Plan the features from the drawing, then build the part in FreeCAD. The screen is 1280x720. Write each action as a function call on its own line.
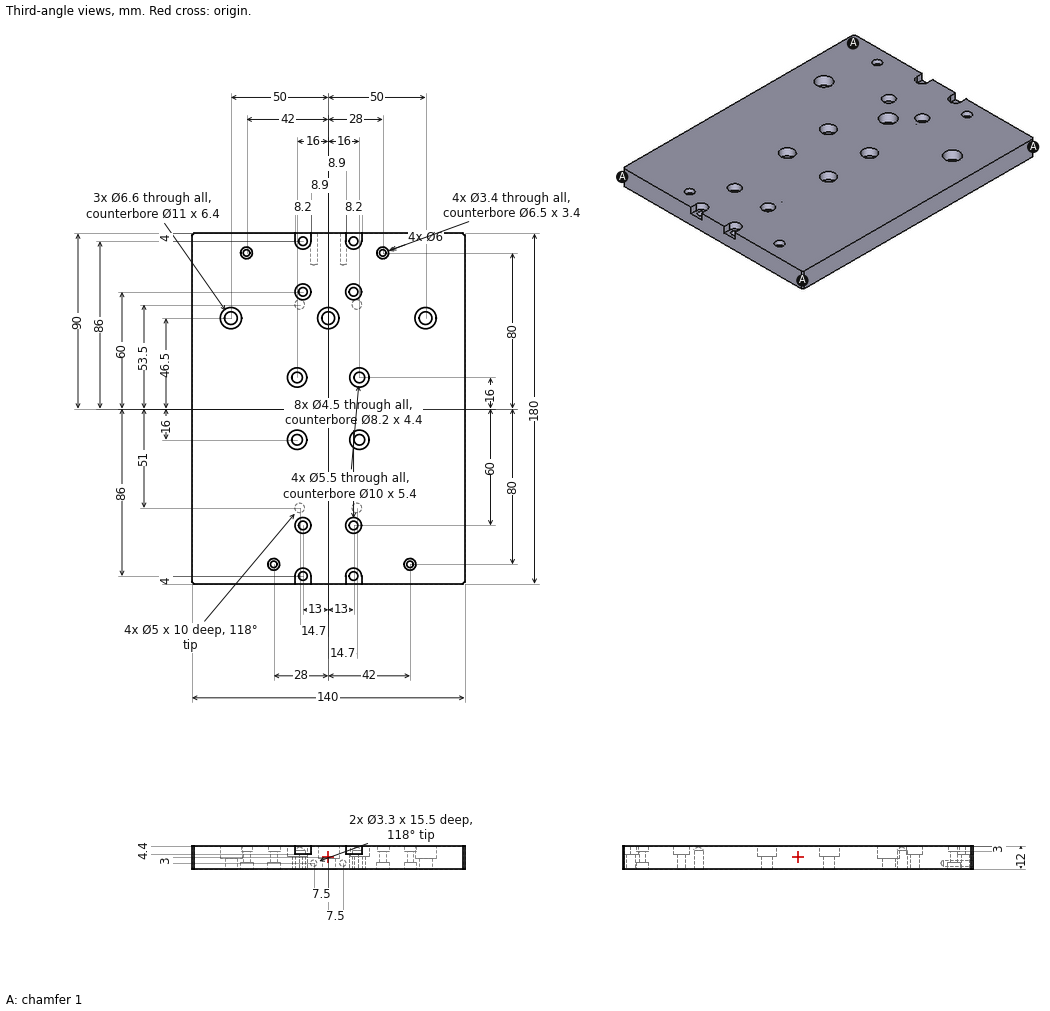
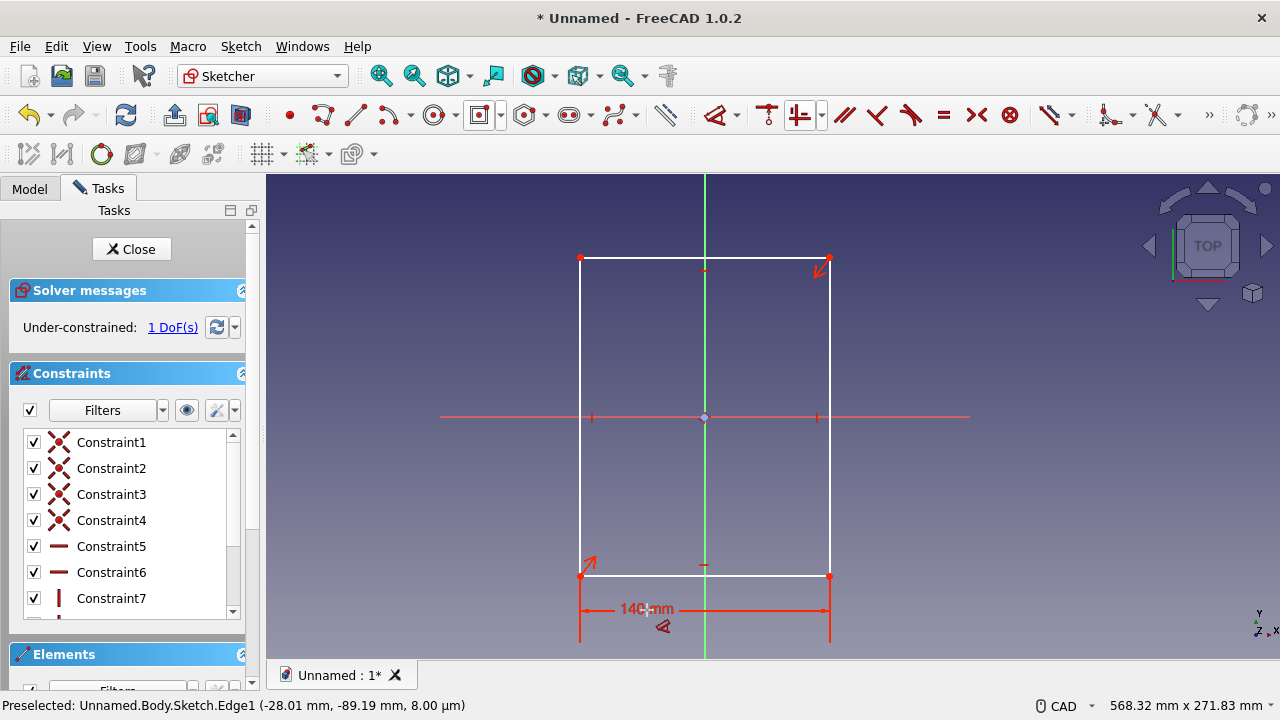
click(830, 481)
click(864, 344)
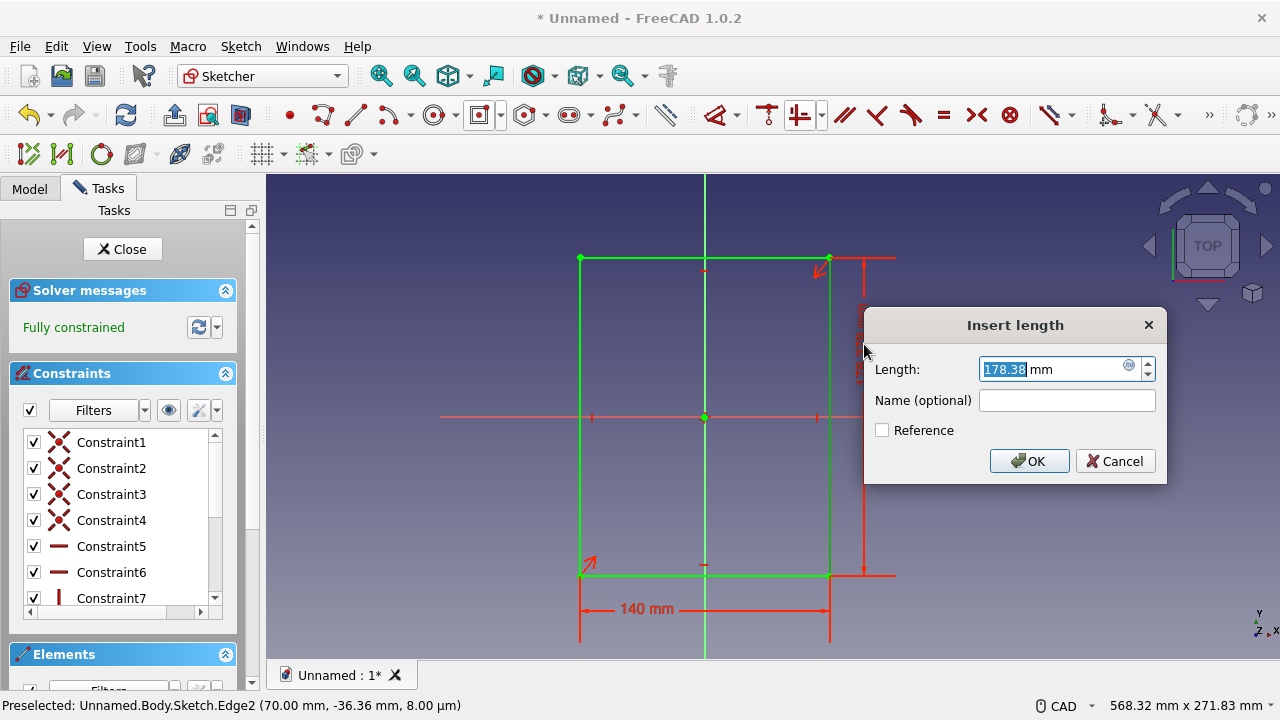
text(180)
key(Return)
key(Escape)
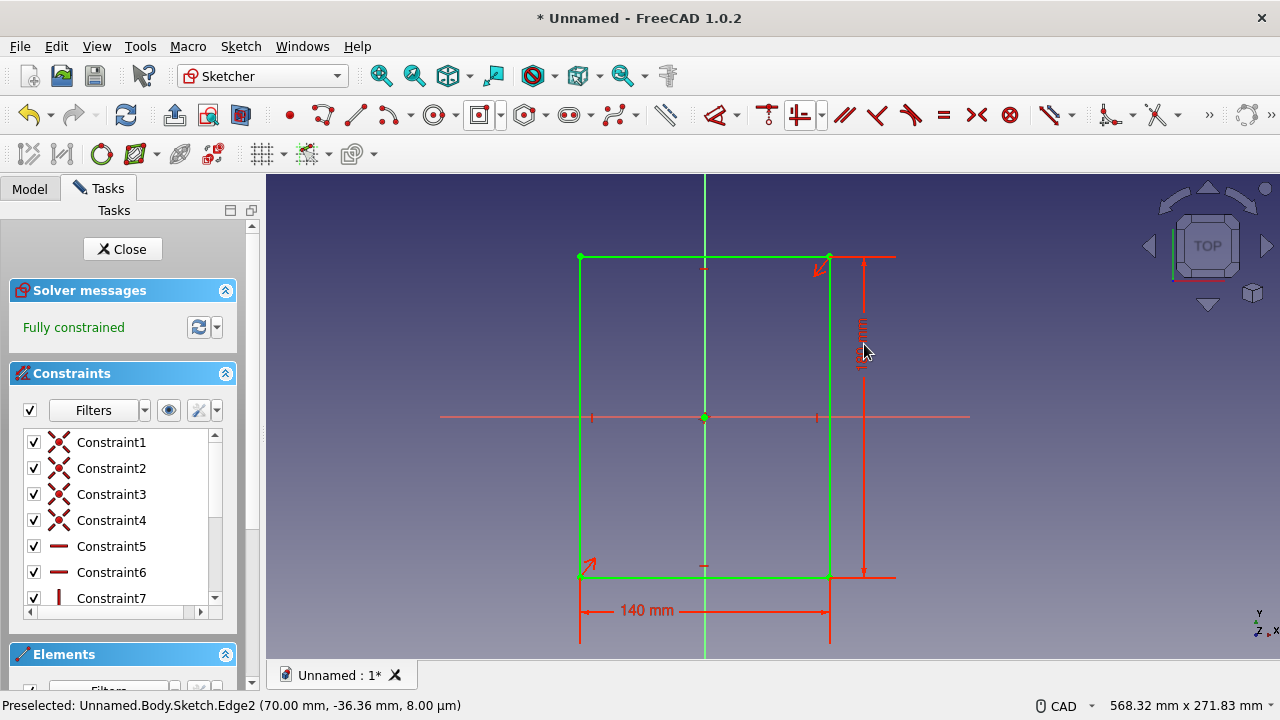
click(123, 249)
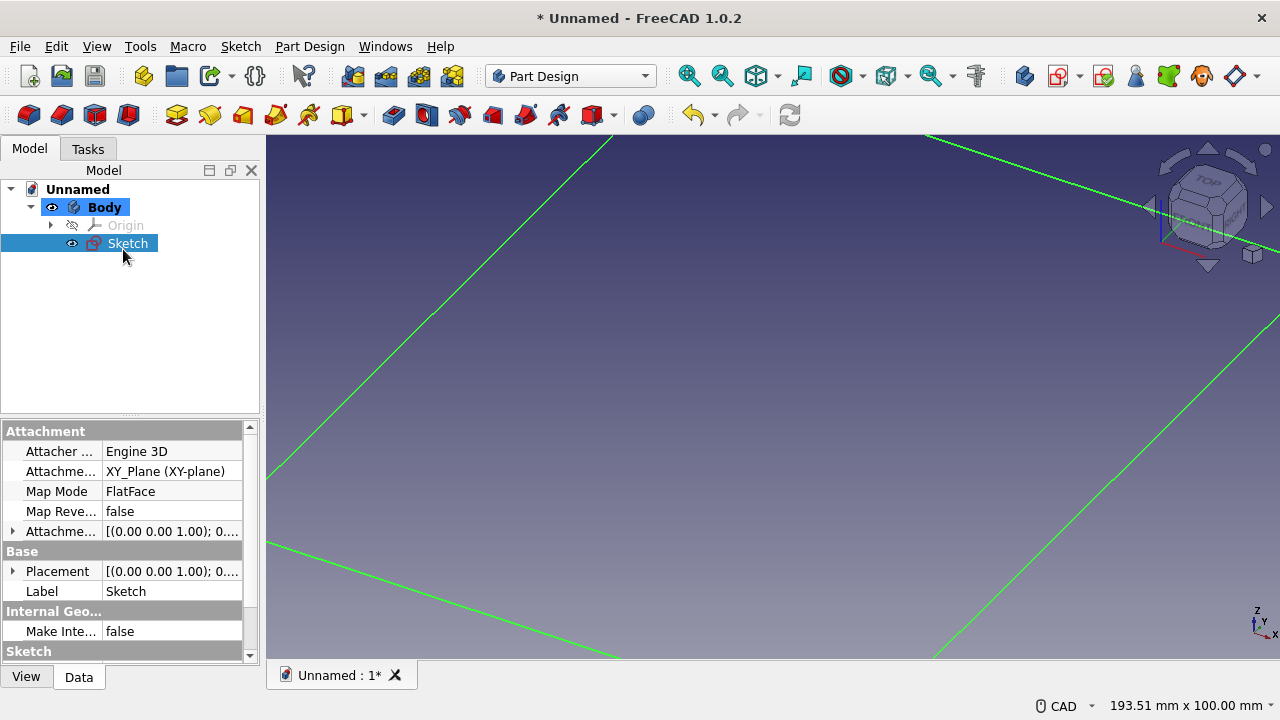
click(177, 116)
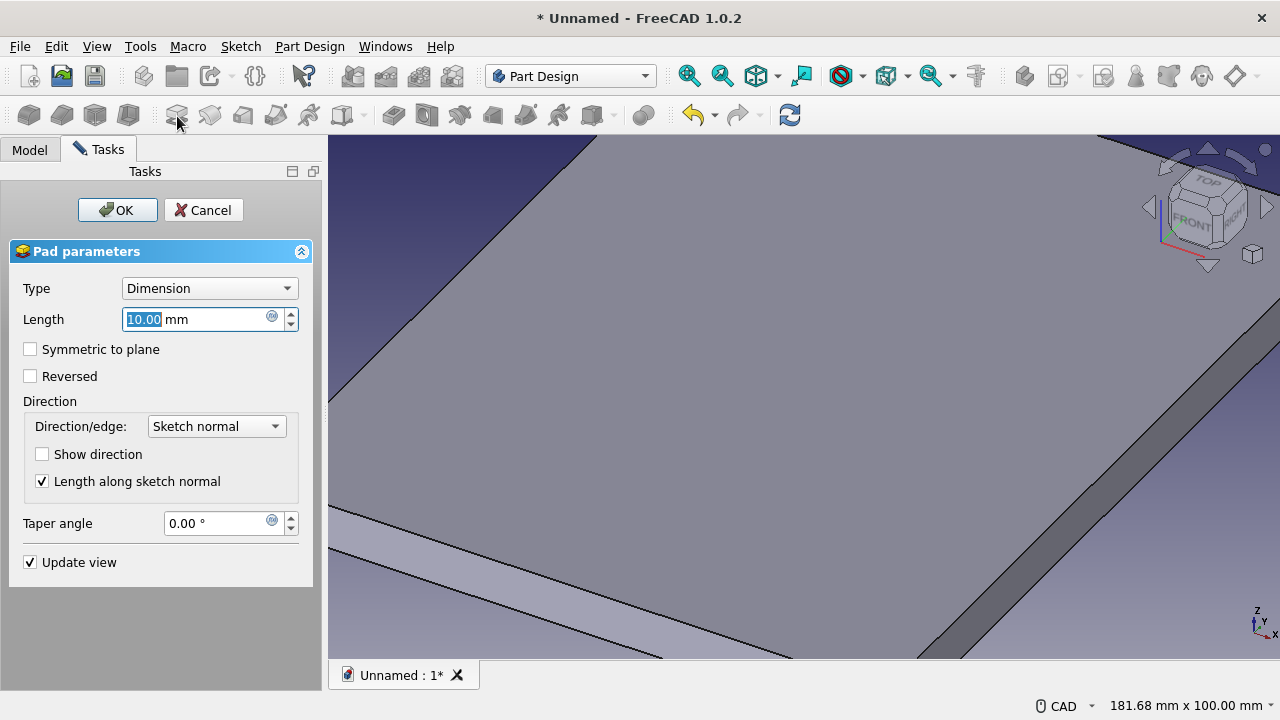
text(12)
key(Tab)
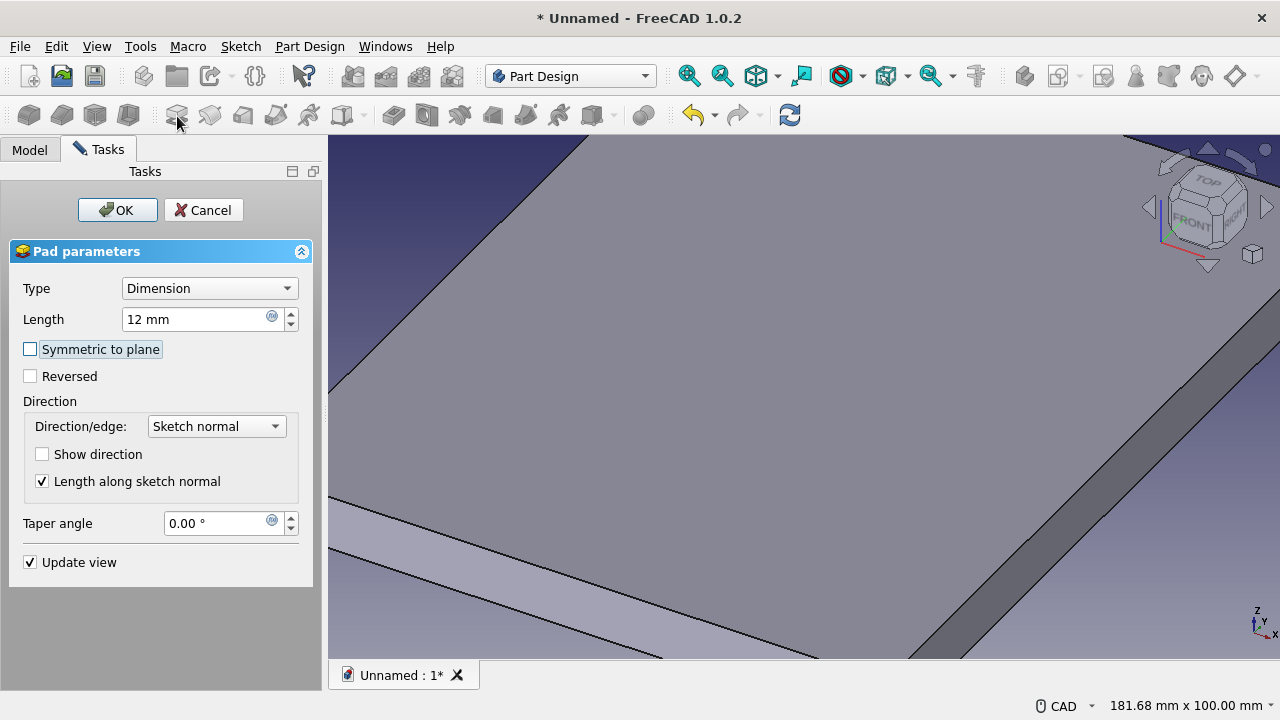
click(31, 349)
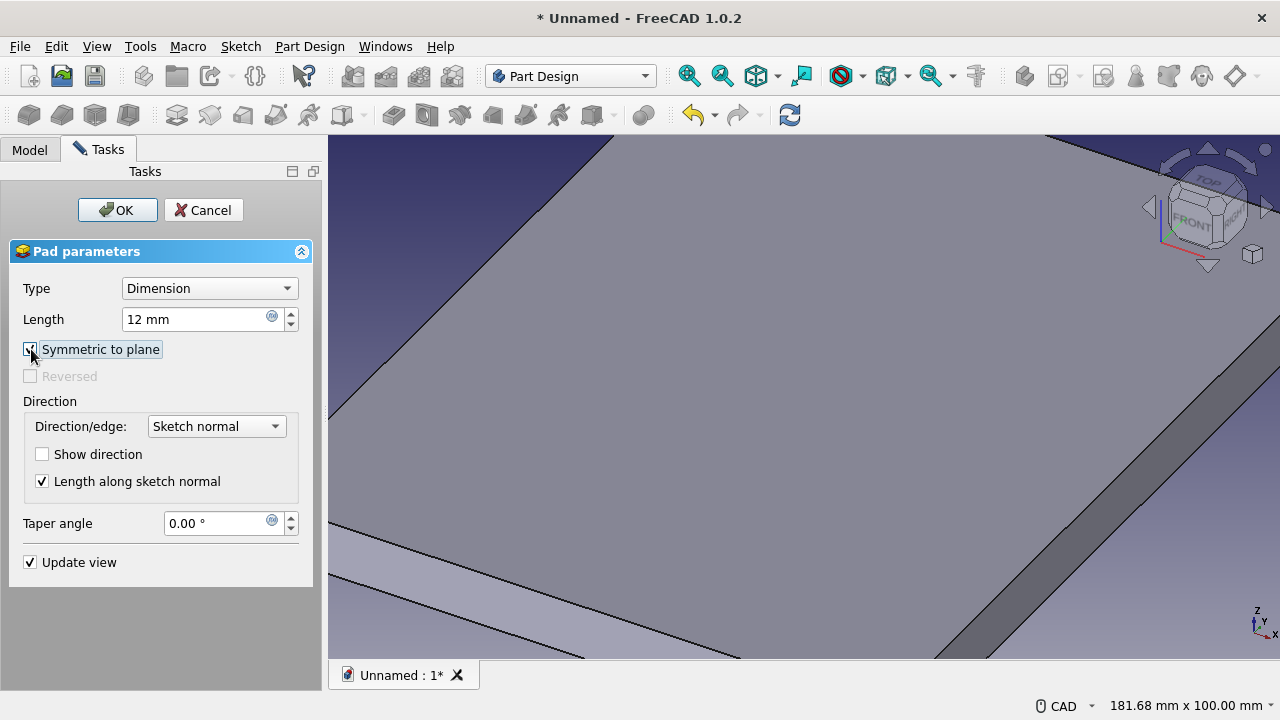
click(118, 210)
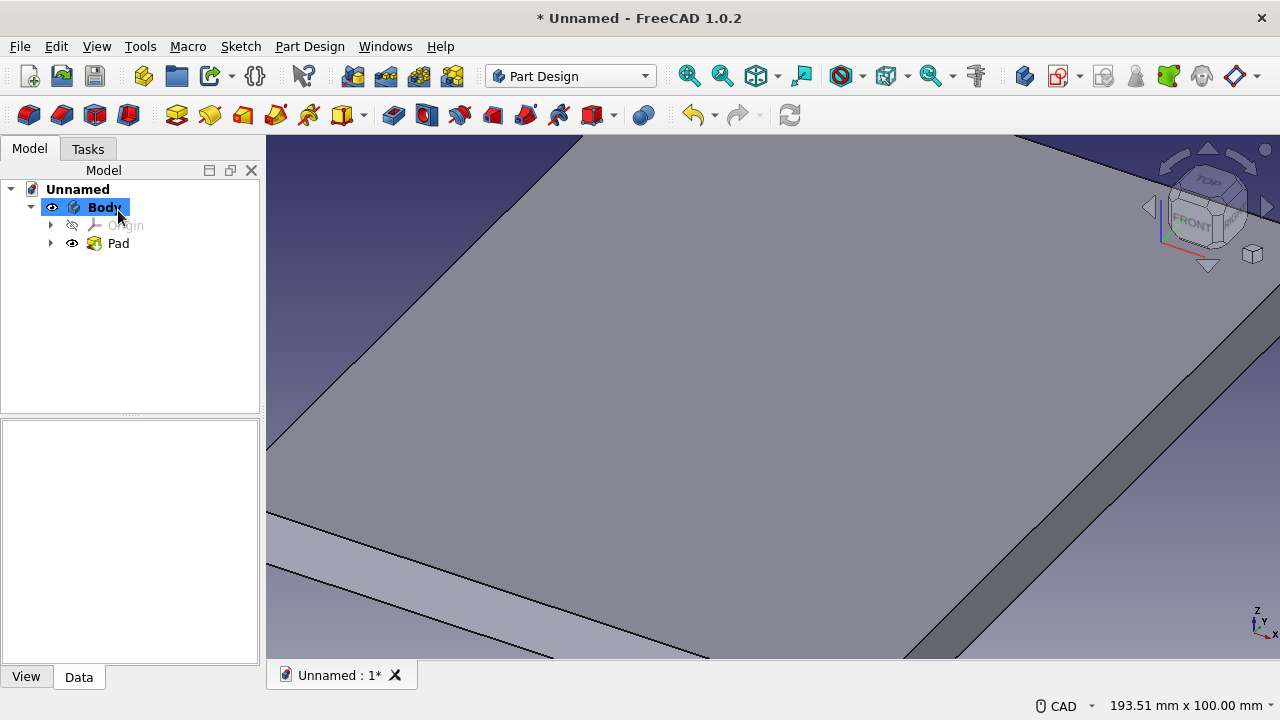
click(690, 76)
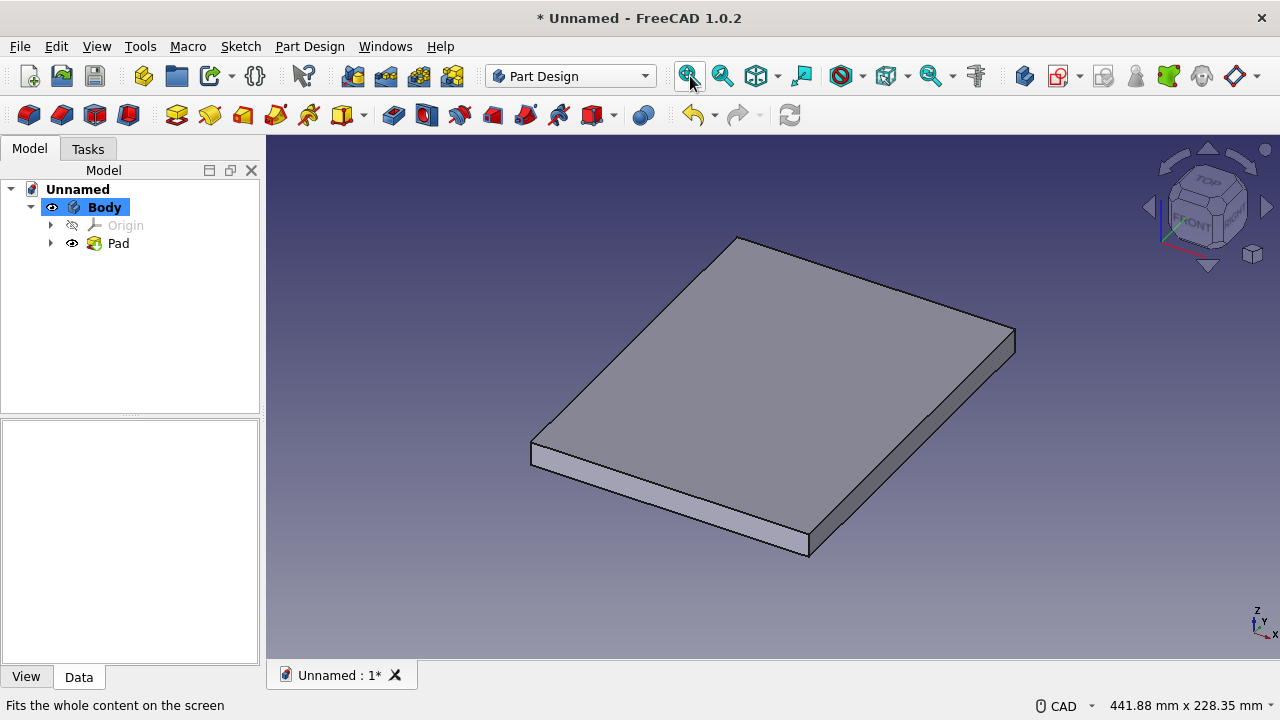
click(773, 385)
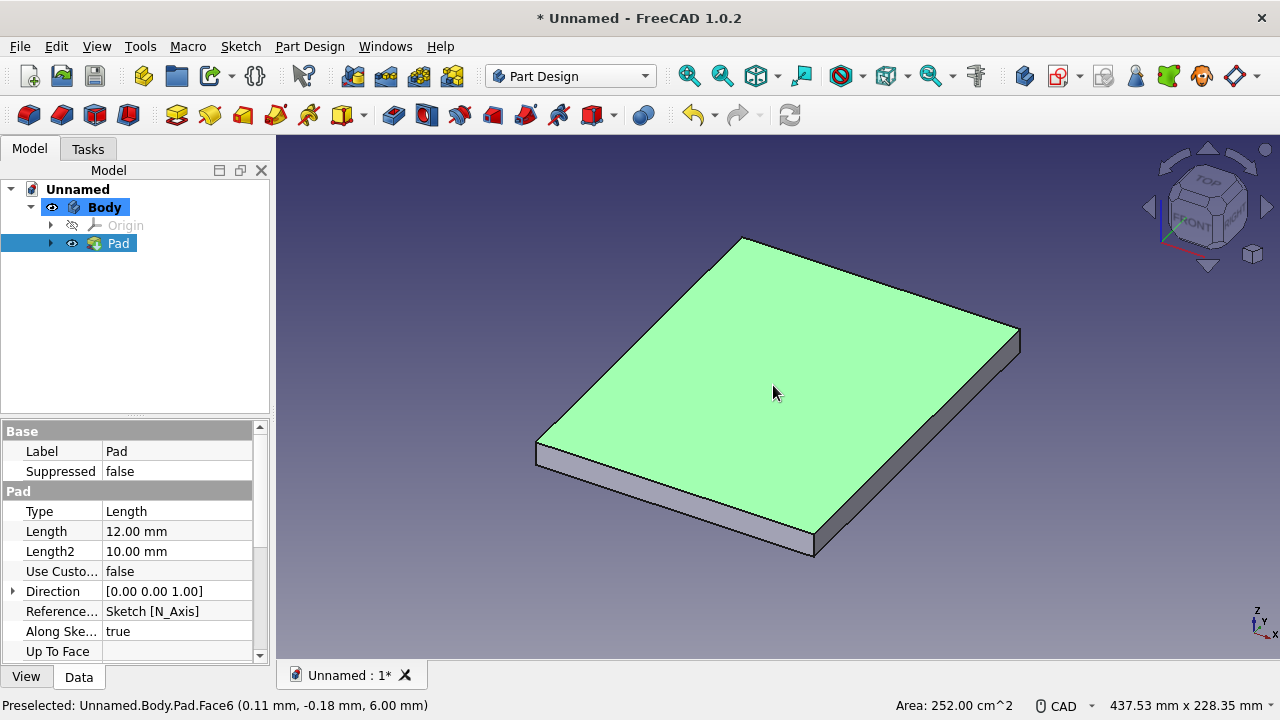
click(1058, 76)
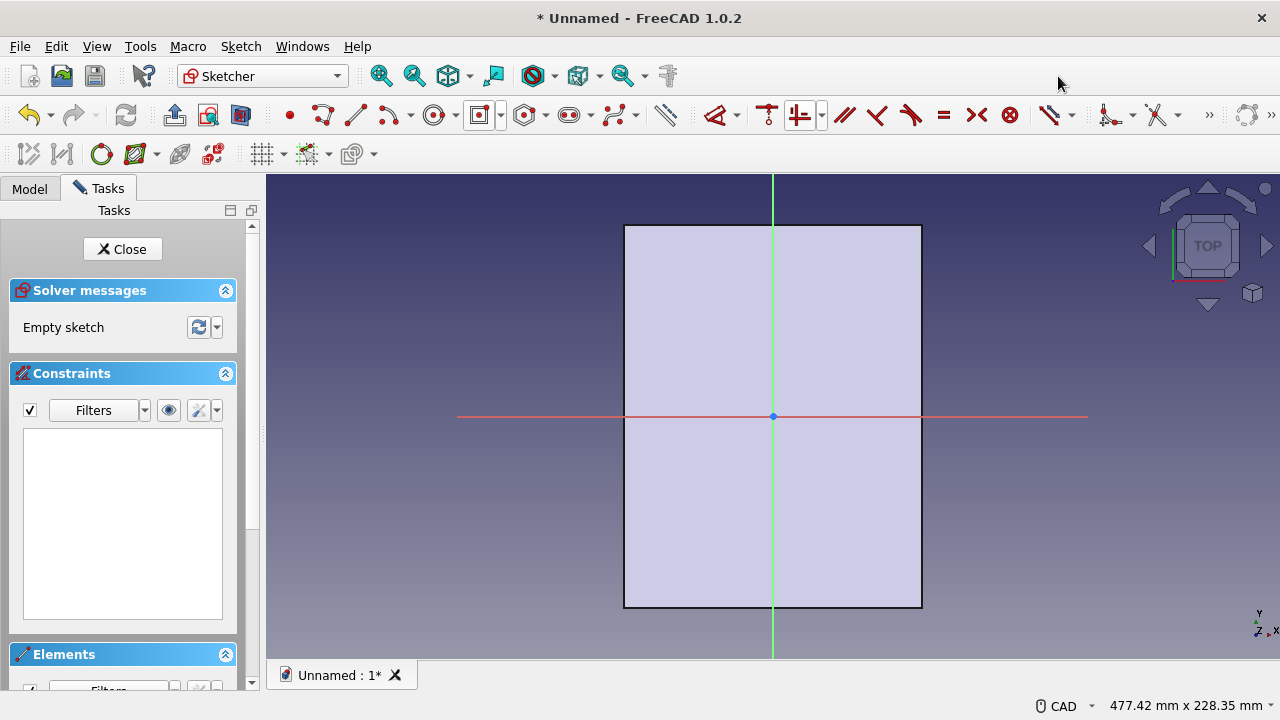
click(434, 116)